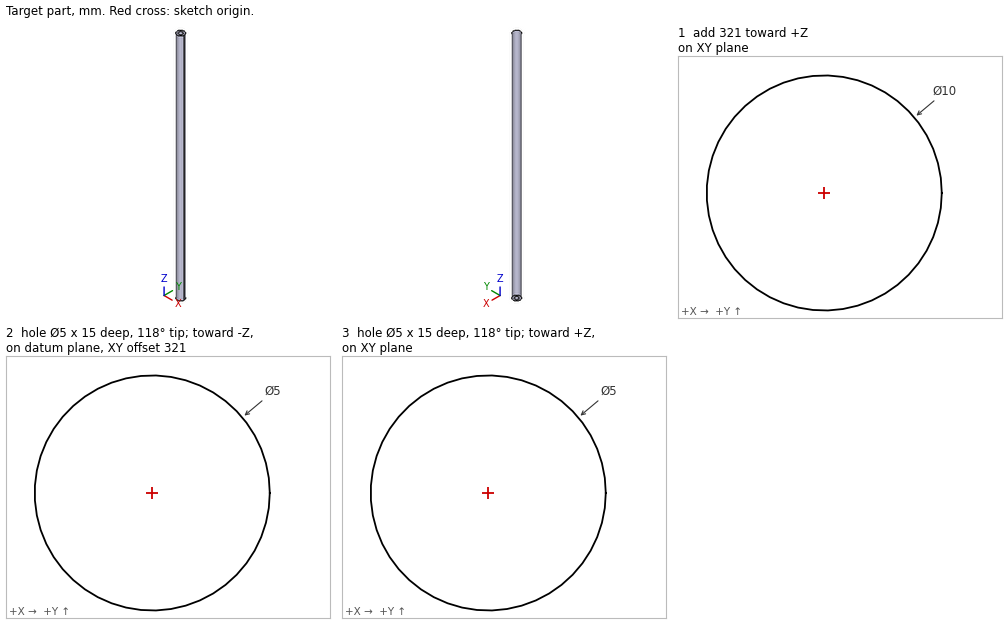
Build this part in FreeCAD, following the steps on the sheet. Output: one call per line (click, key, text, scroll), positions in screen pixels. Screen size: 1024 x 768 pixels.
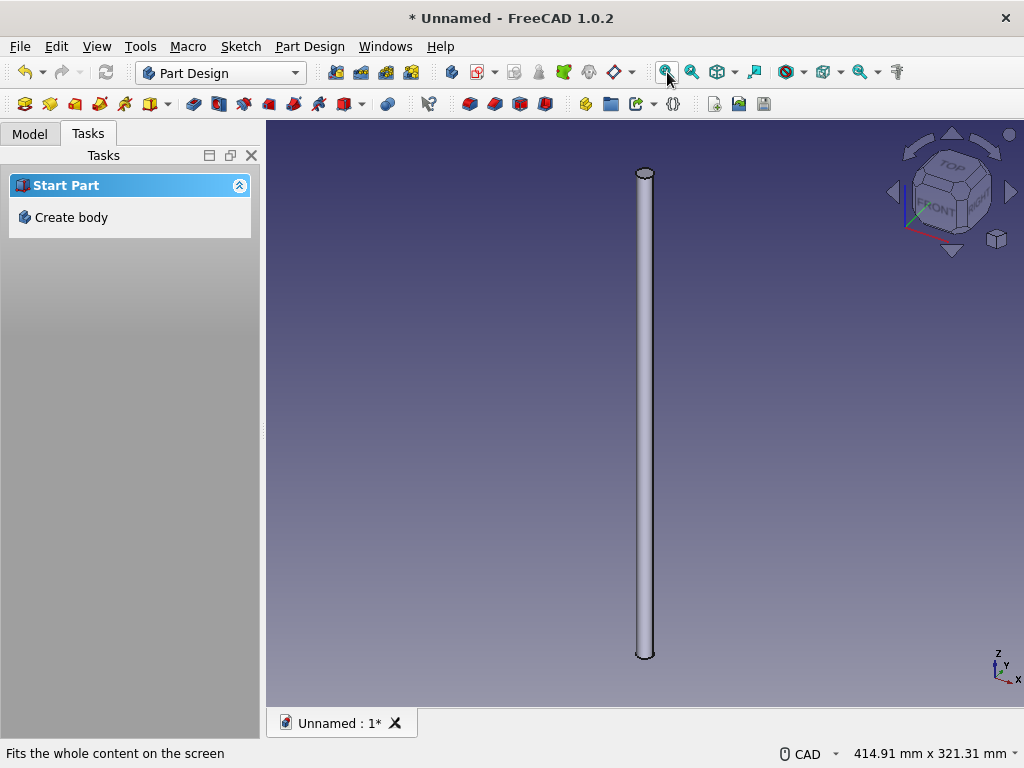
key(0)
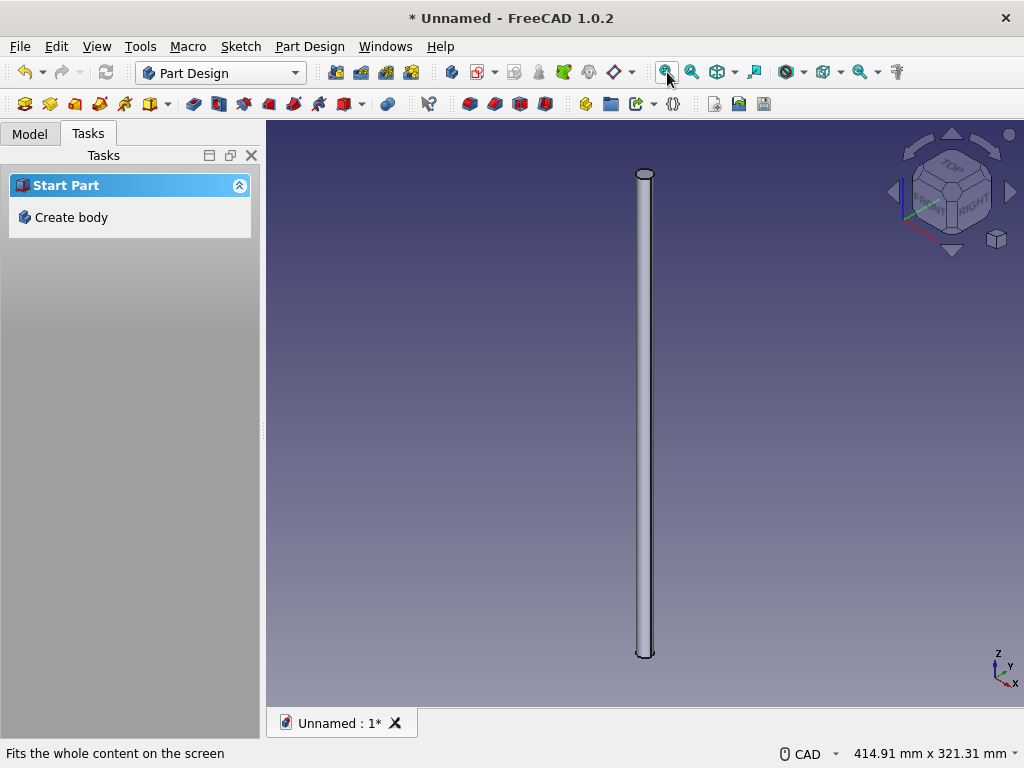
key(2)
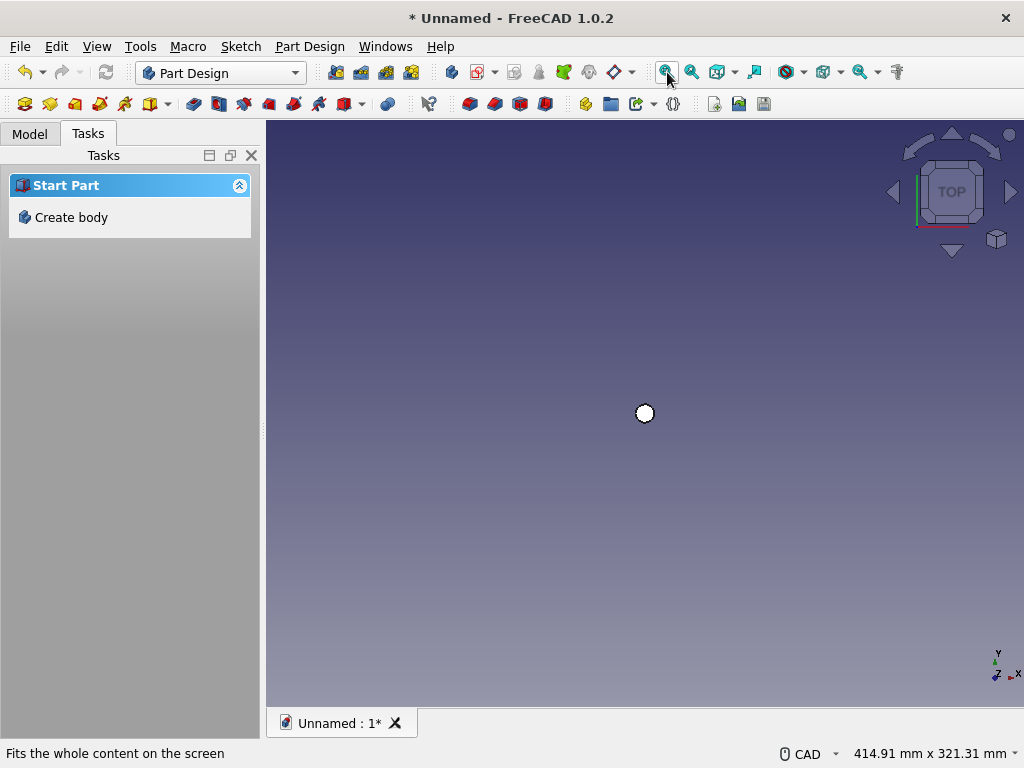
click(667, 72)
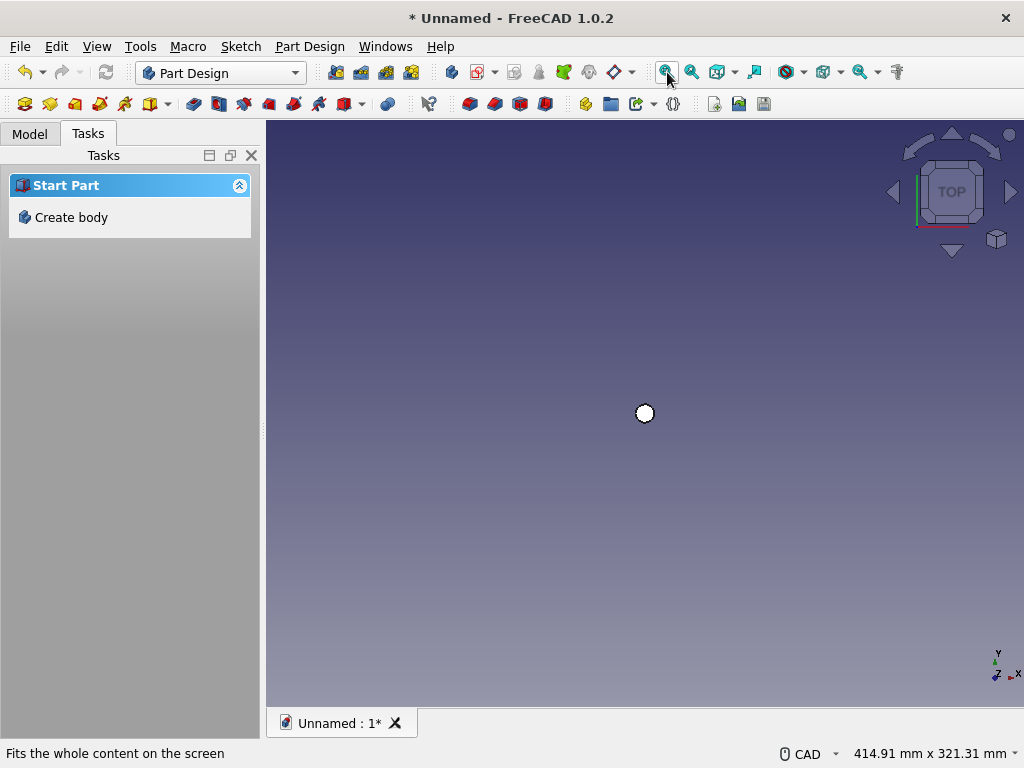
key(1)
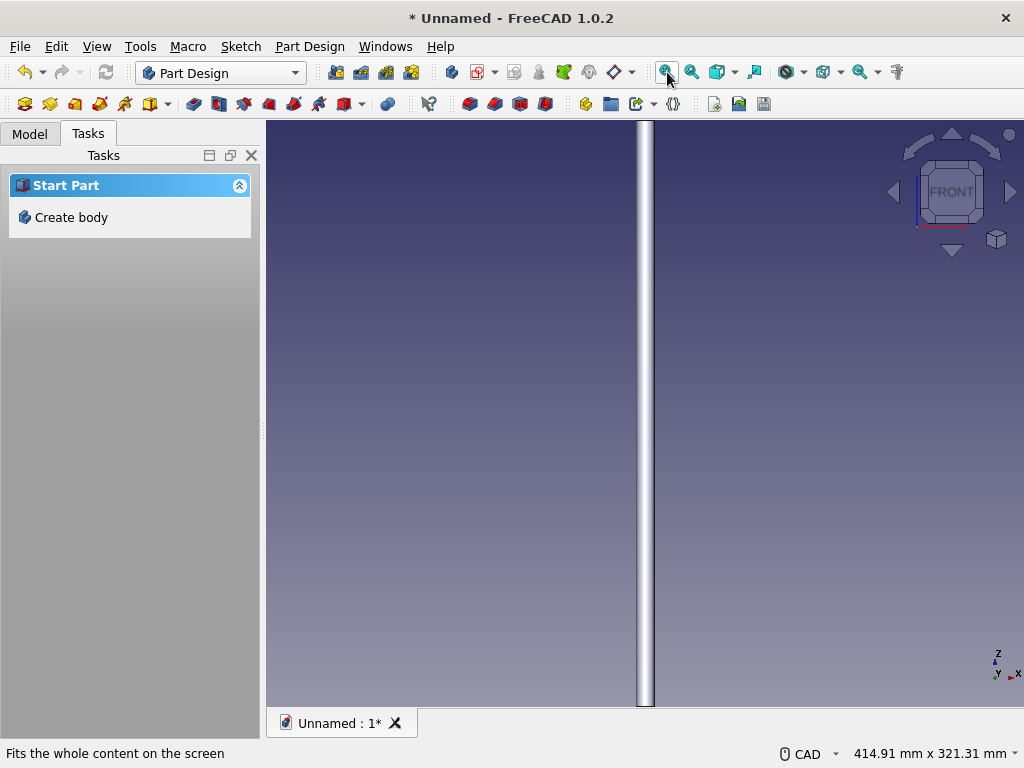
click(667, 72)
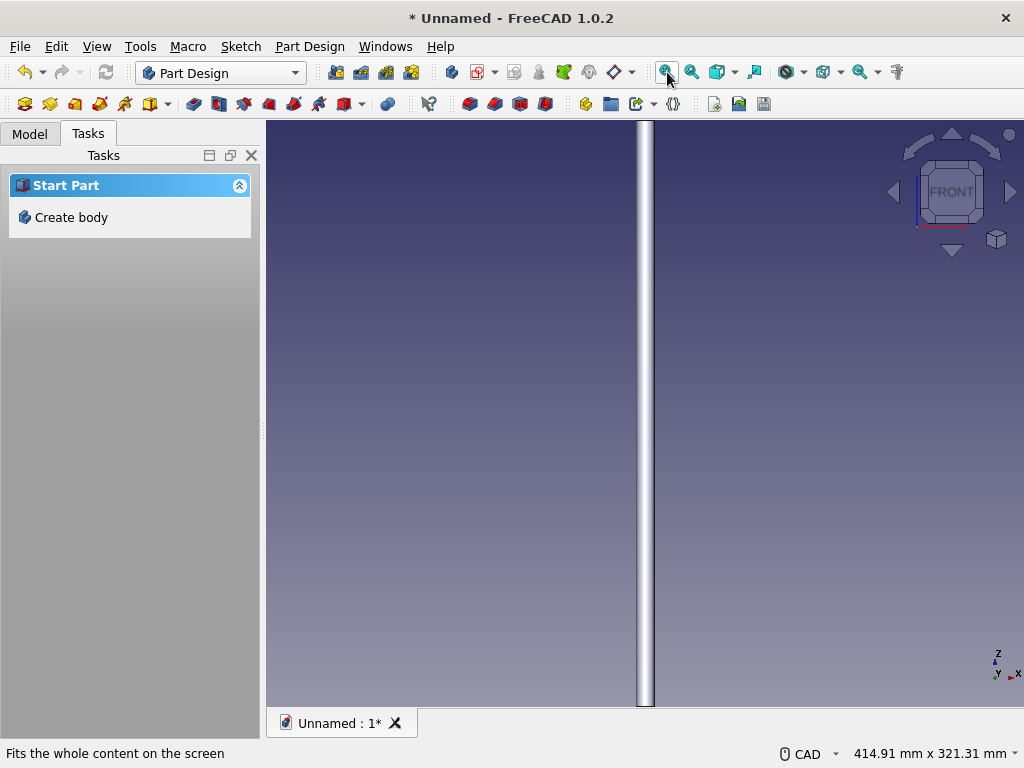
click(30, 134)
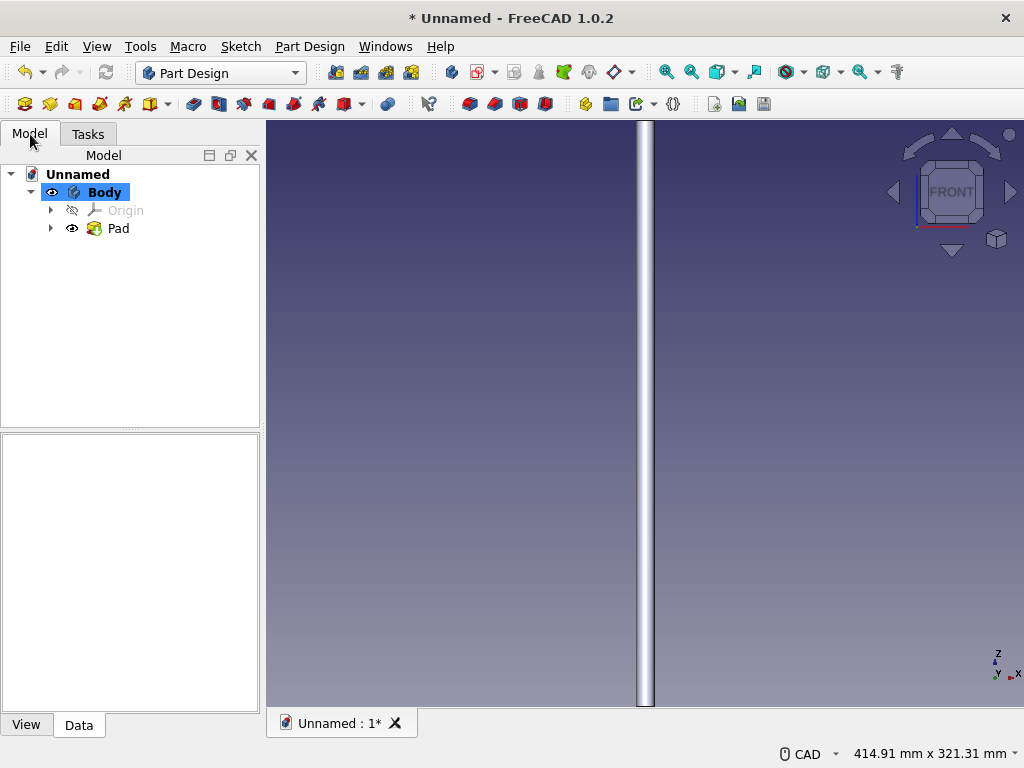
click(51, 210)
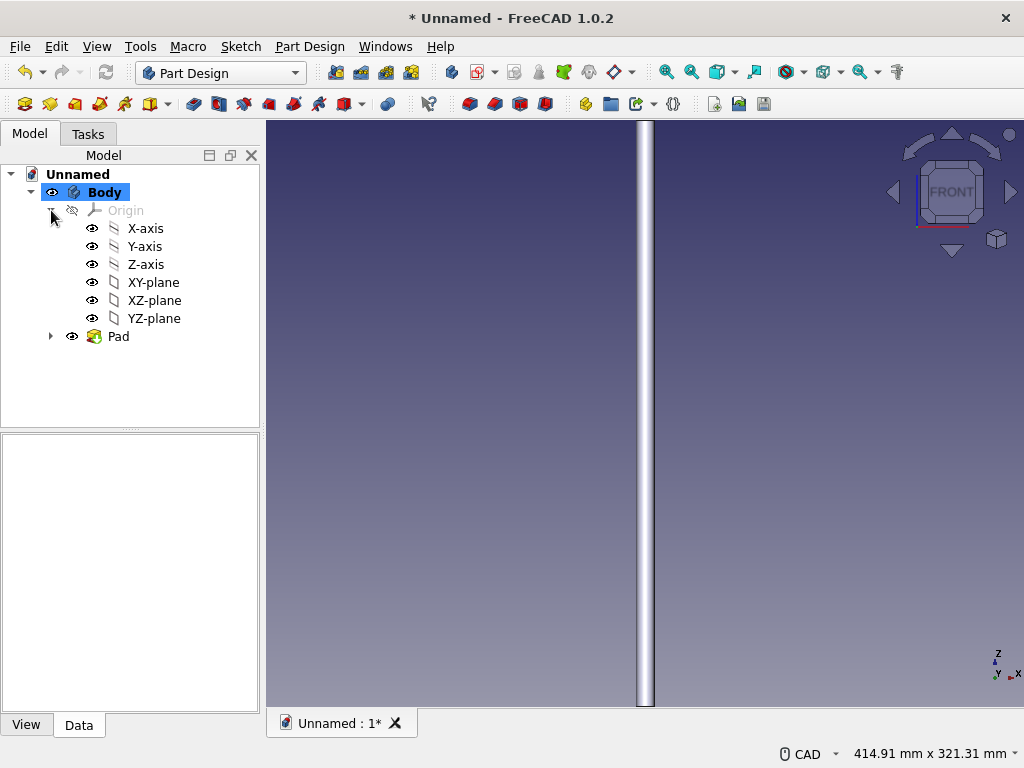
click(137, 282)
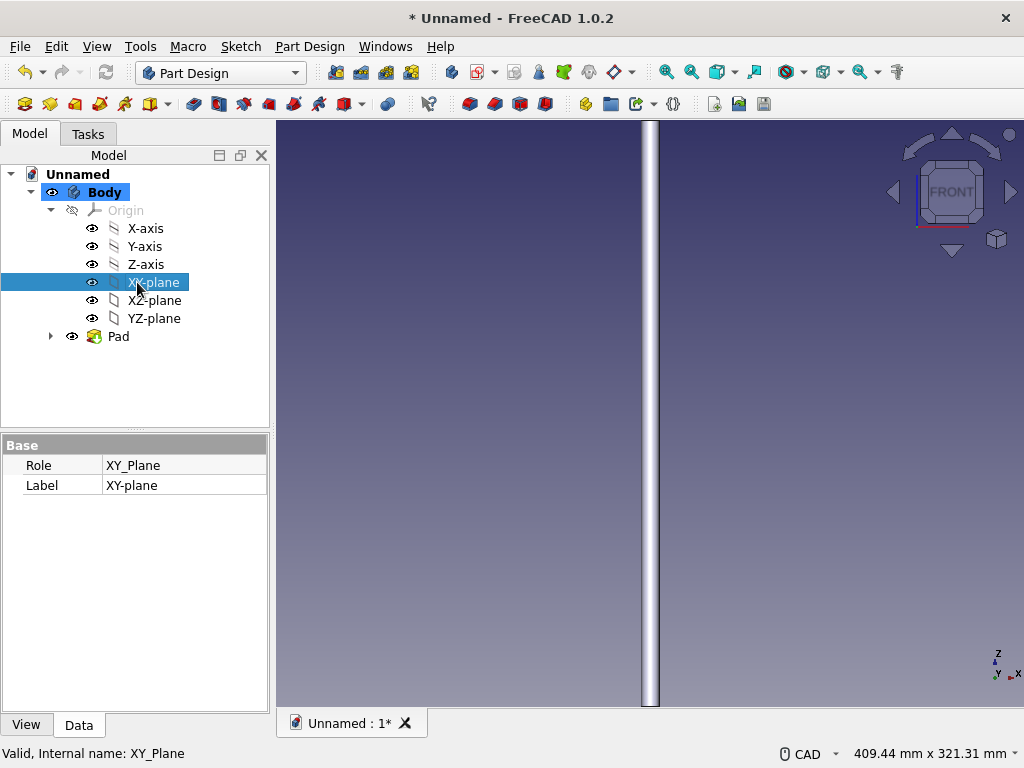
click(614, 72)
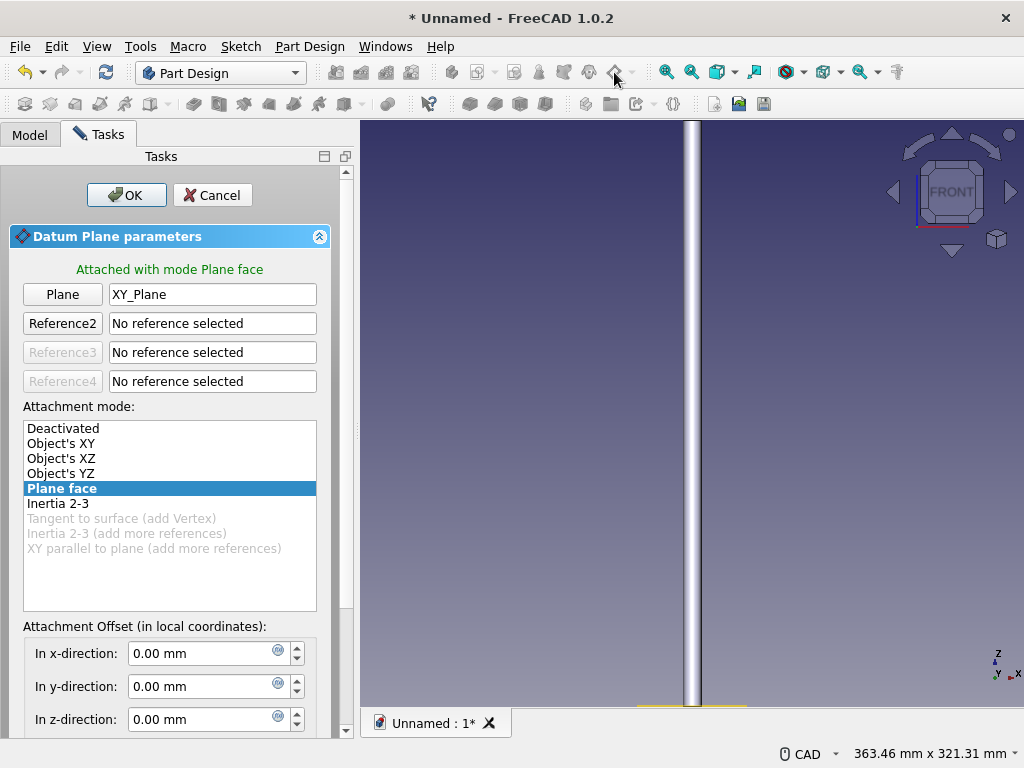
triple_click(210, 720)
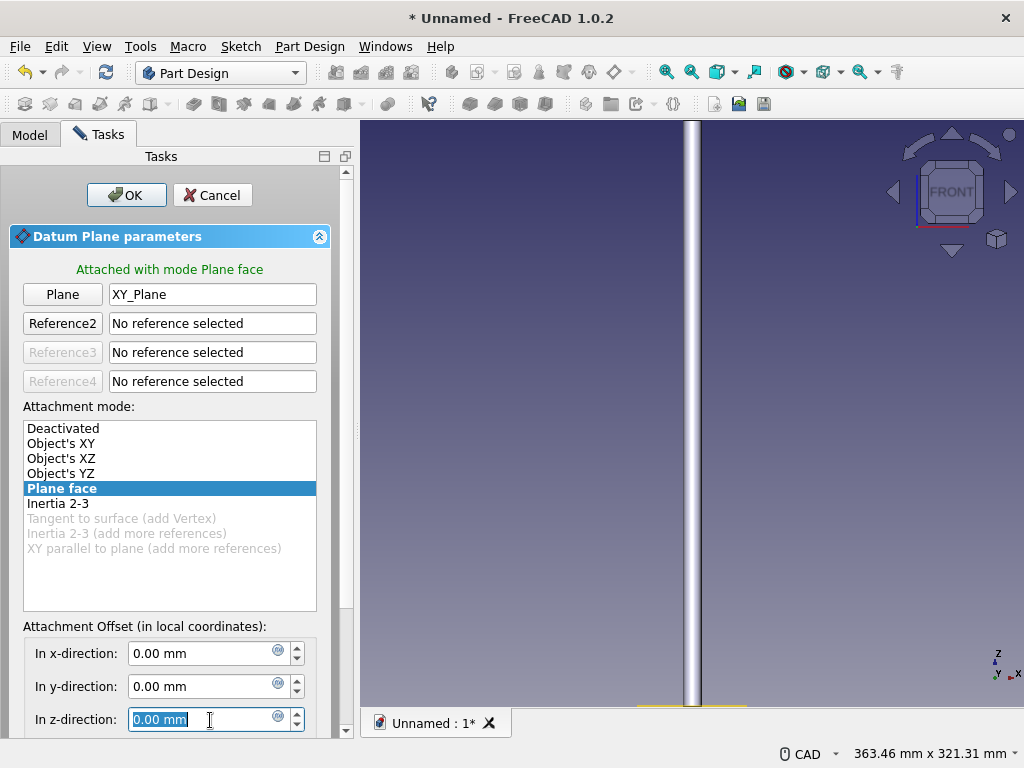
text(321)
key(Tab)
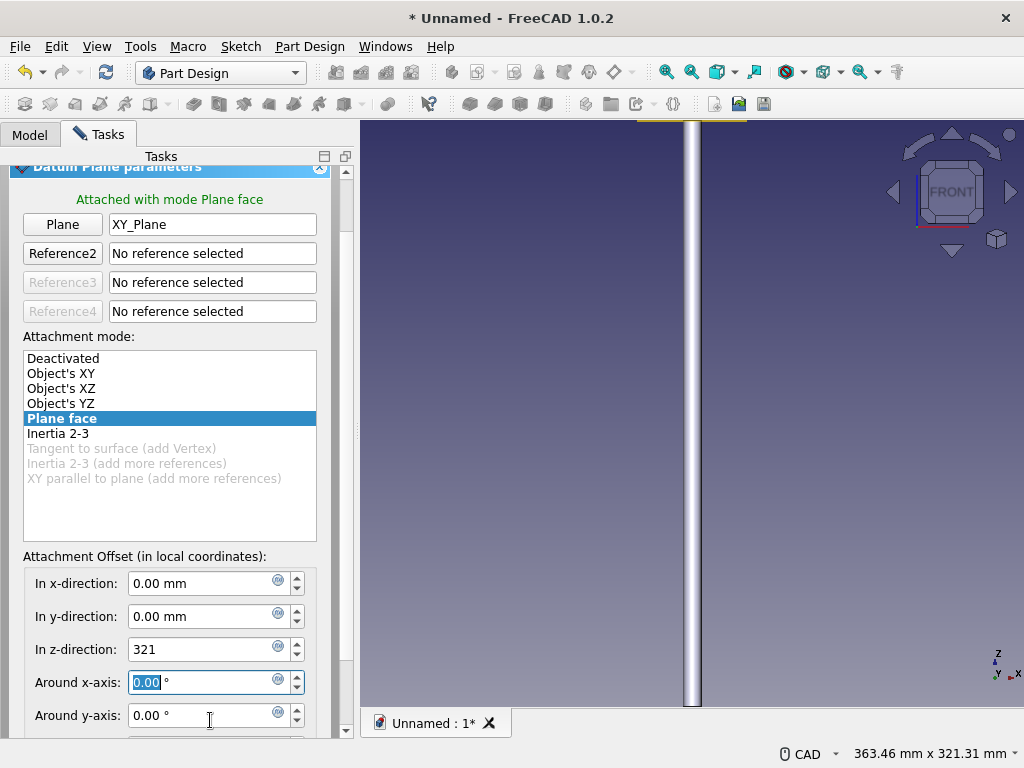
scroll(346, 452, up, 2)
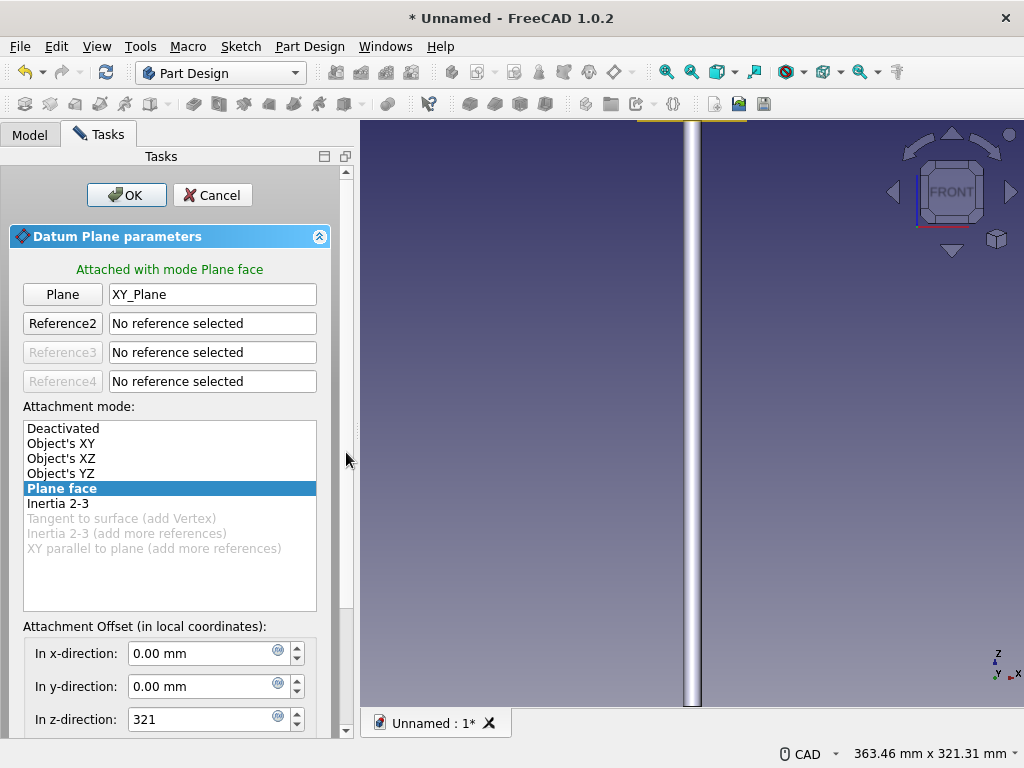
click(127, 195)